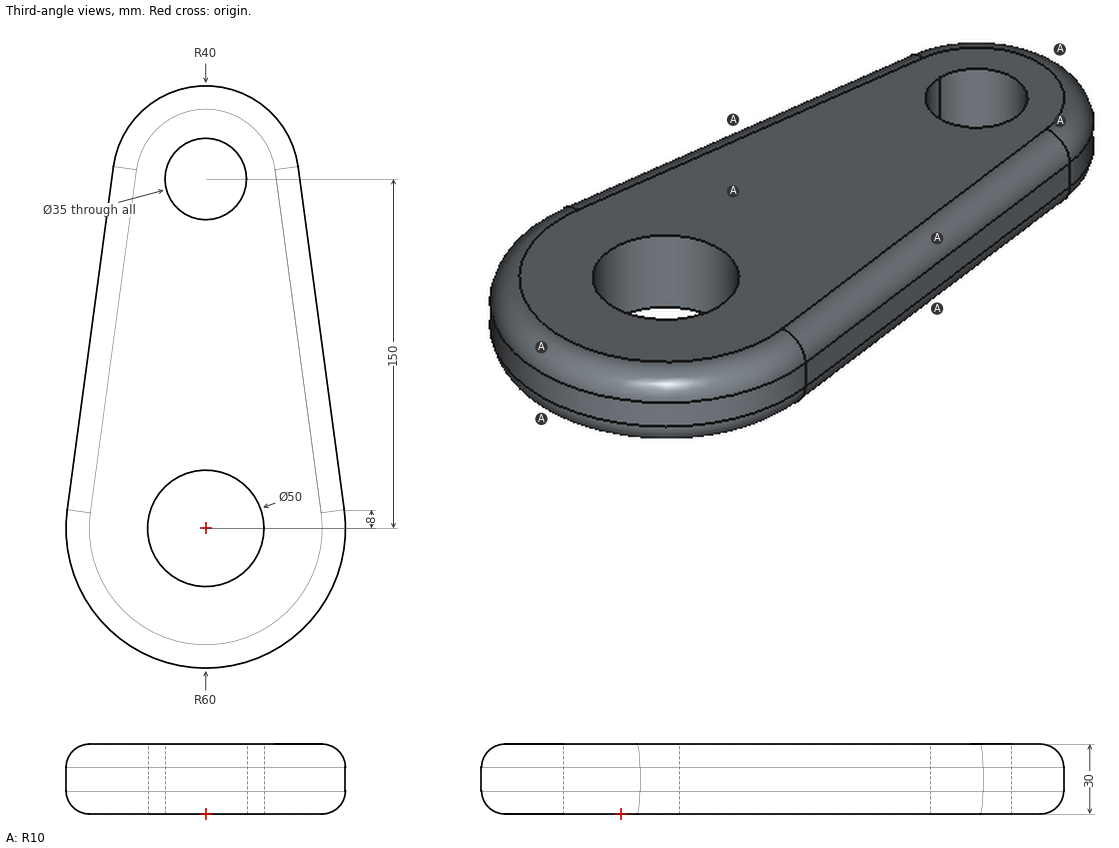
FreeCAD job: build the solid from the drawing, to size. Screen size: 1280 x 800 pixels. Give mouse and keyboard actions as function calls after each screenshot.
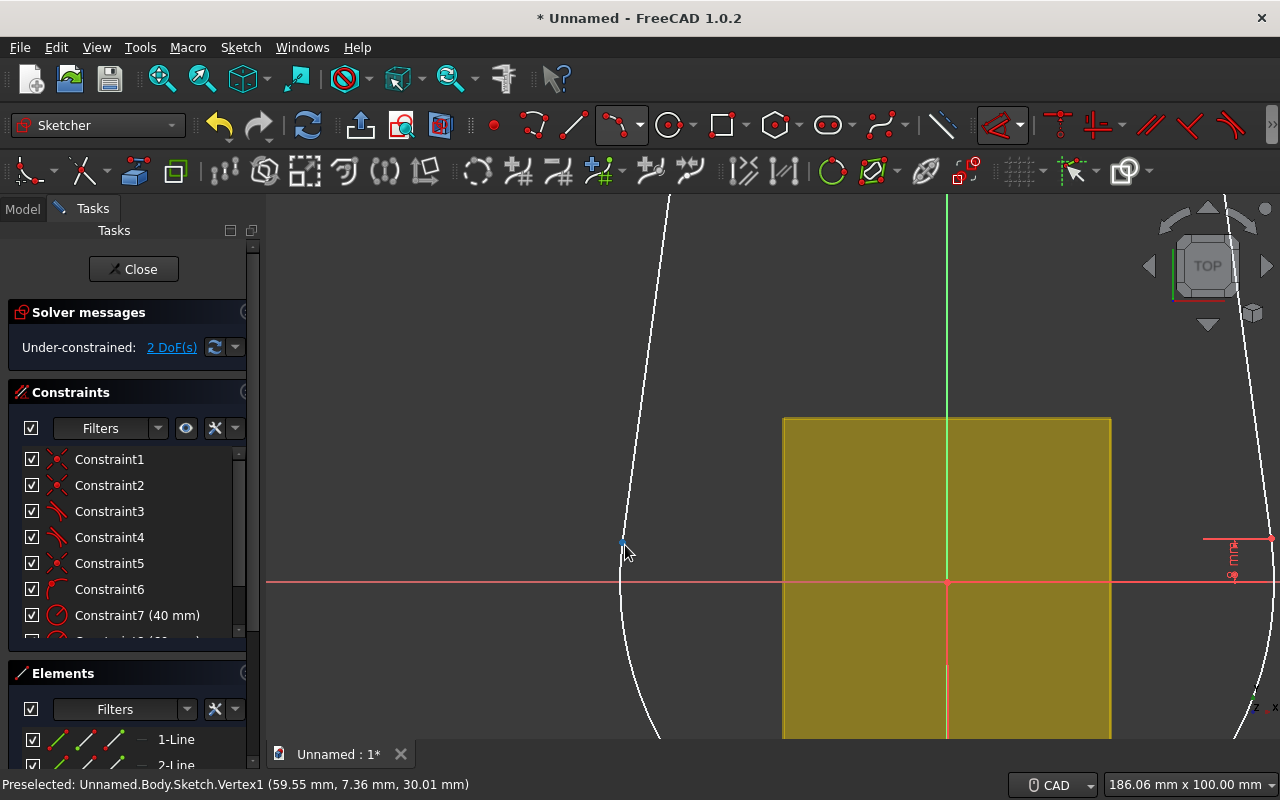
click(623, 542)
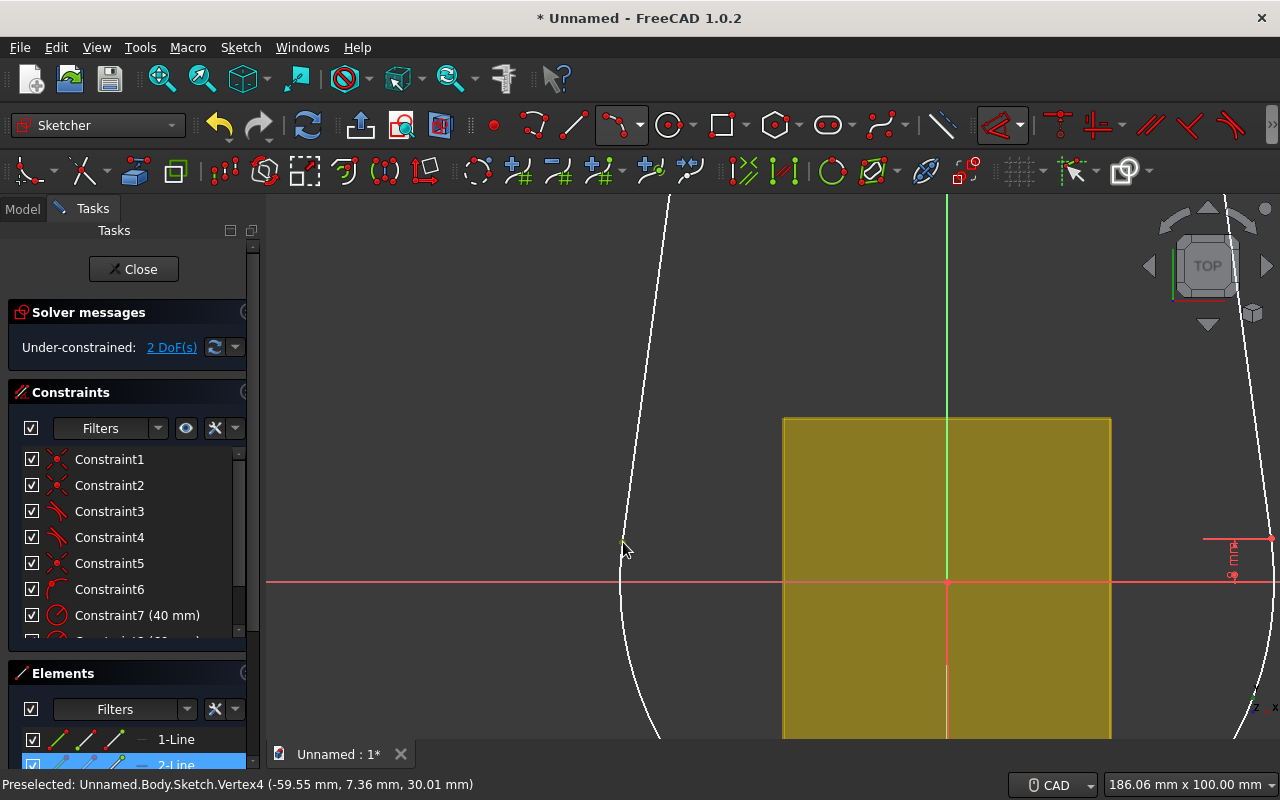
click(1022, 126)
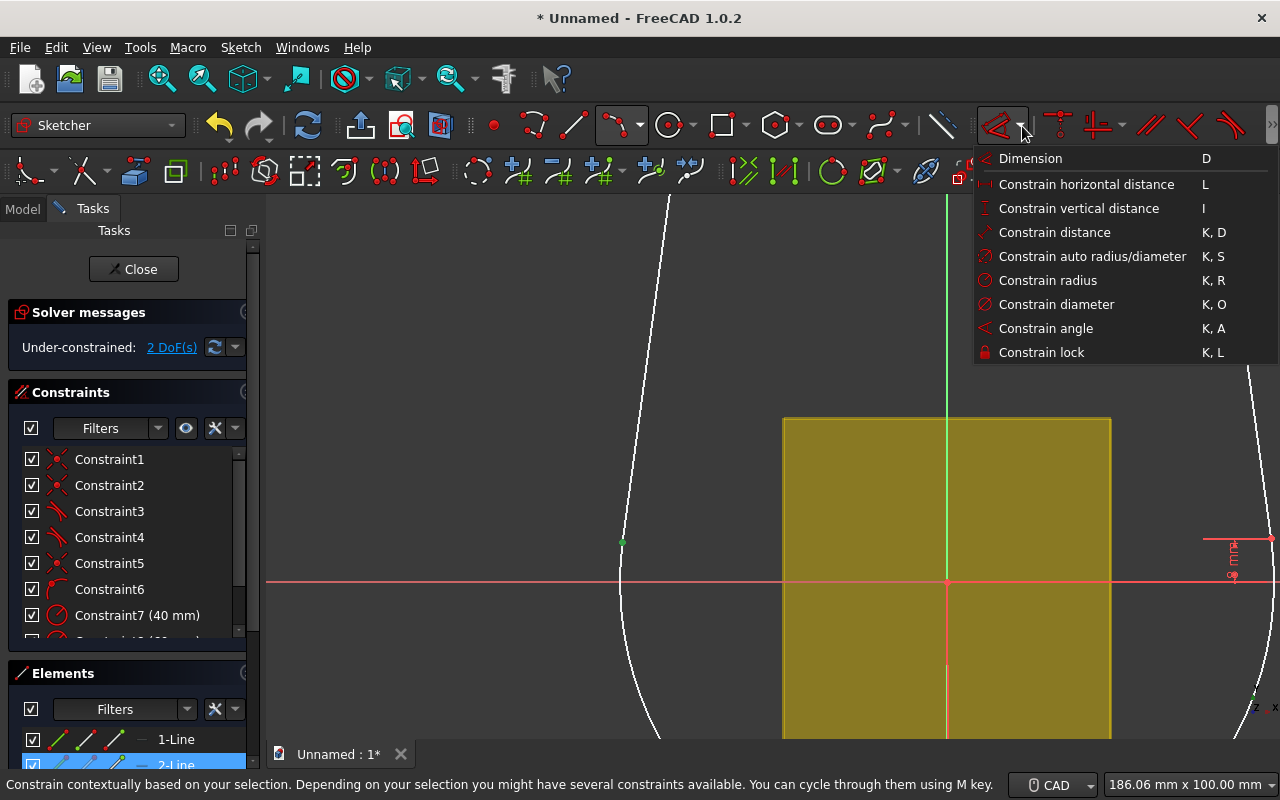
click(1126, 208)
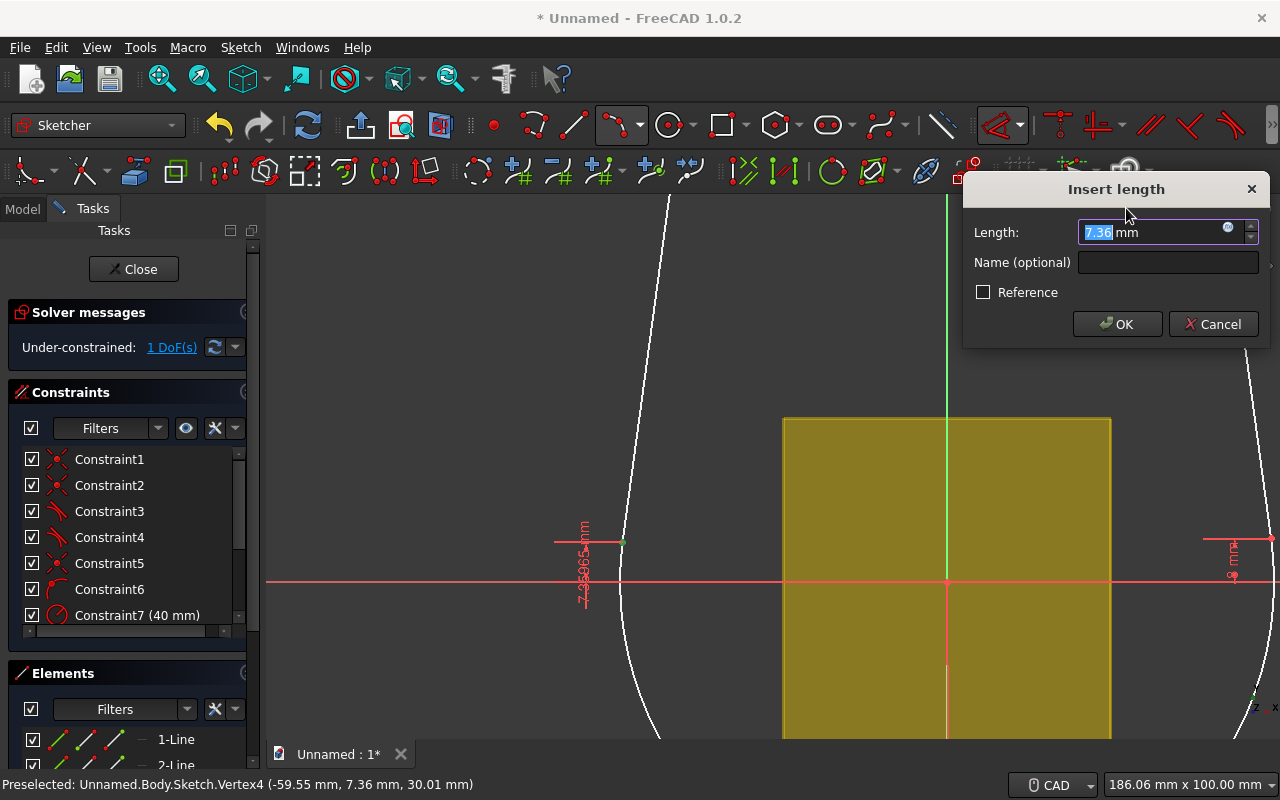
text(8)
key(Return)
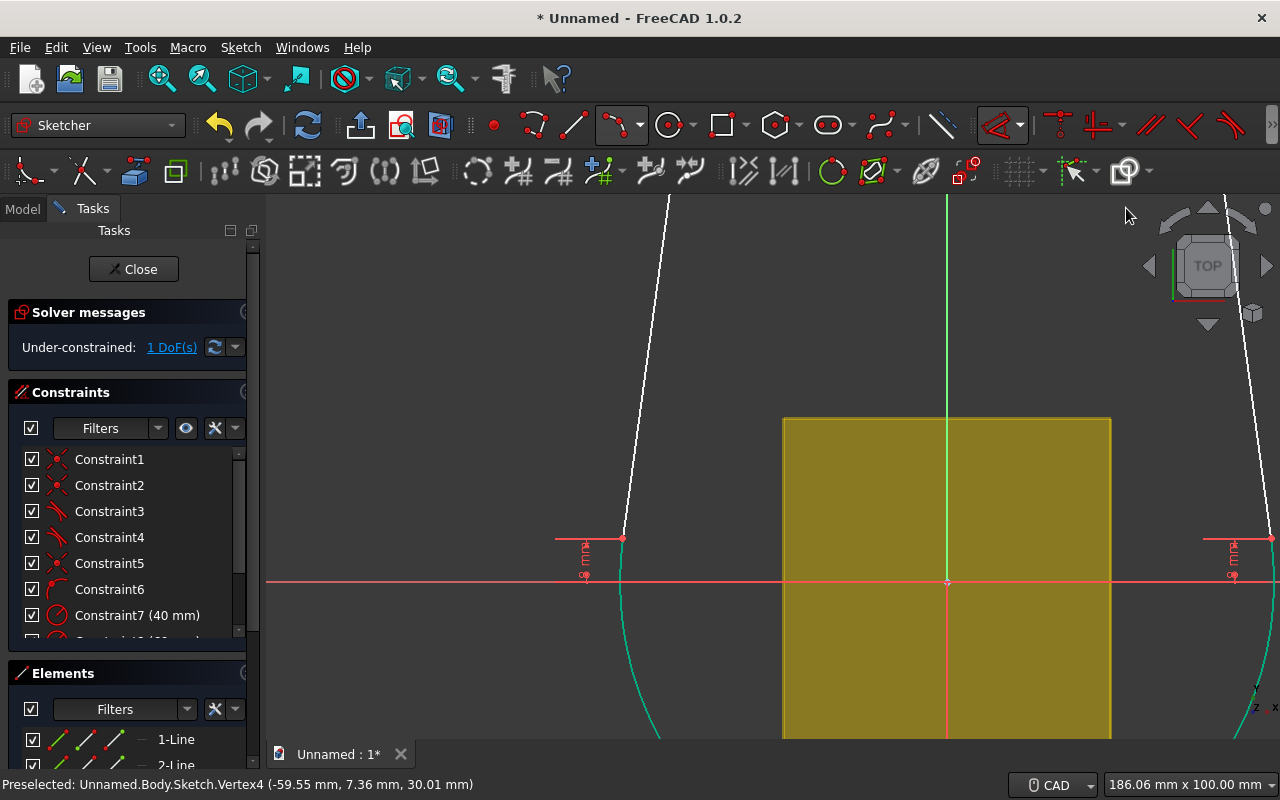
scroll(625, 545, down, 7)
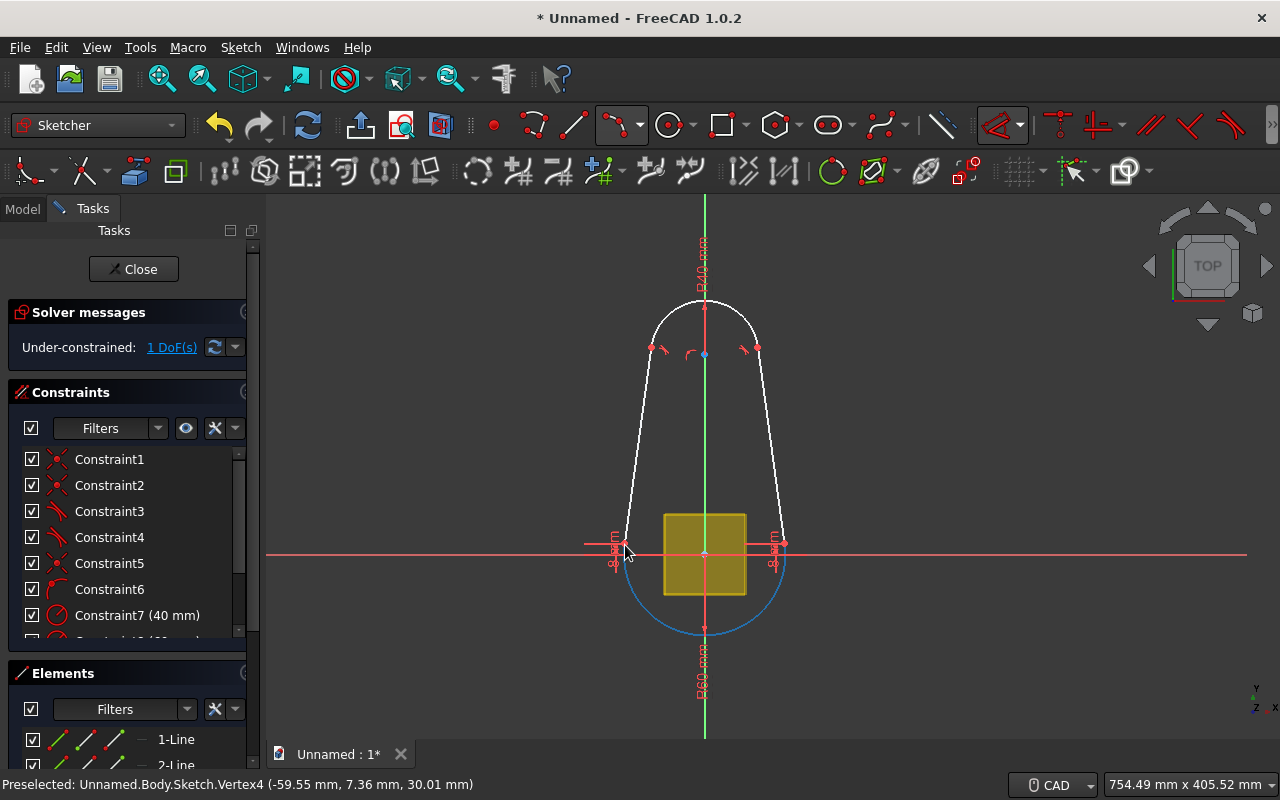
click(705, 355)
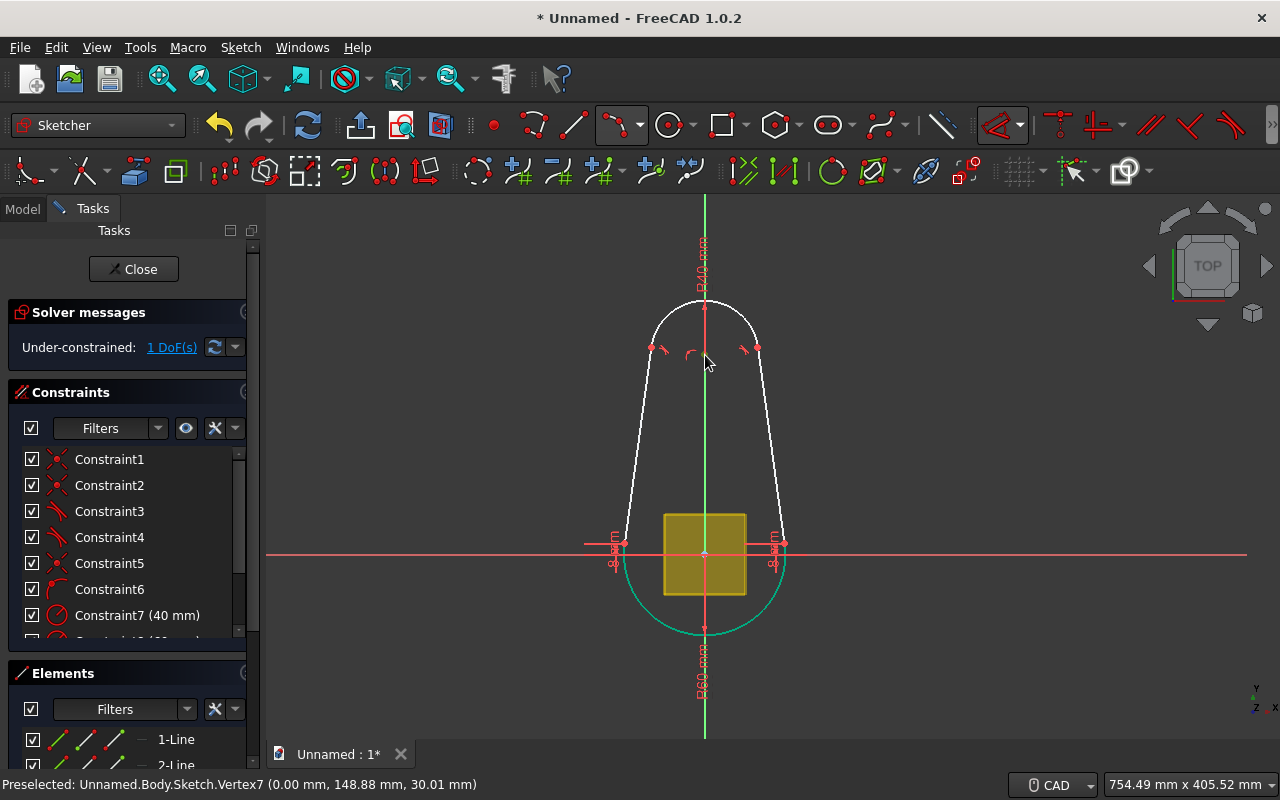
key(i)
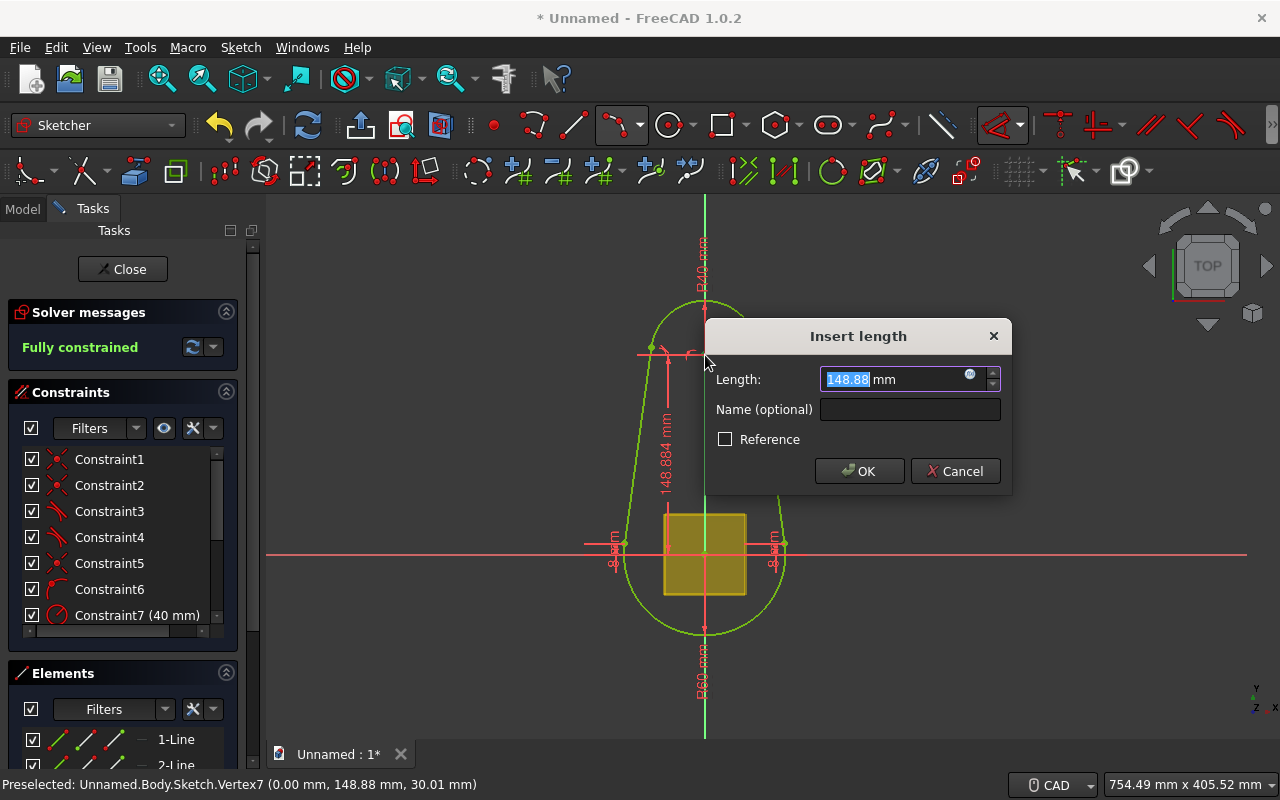
text(150)
key(Return)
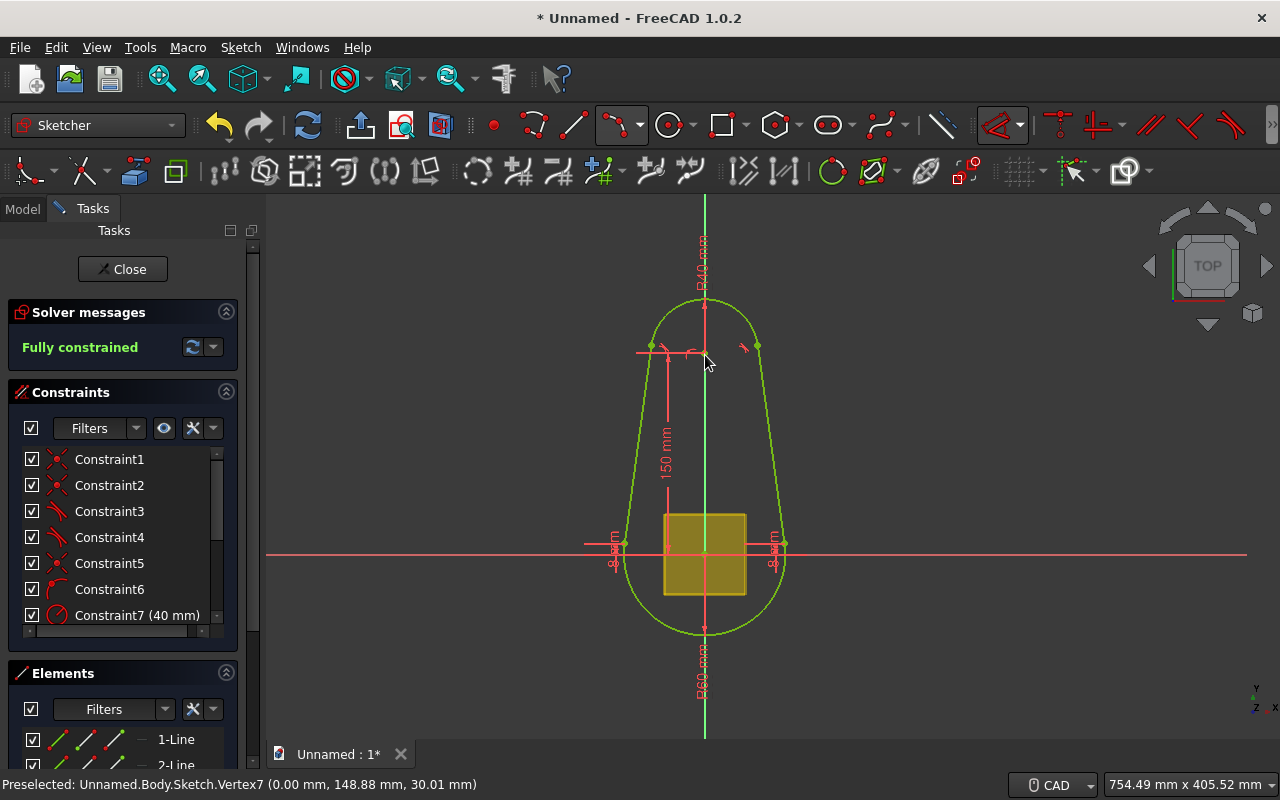
click(123, 269)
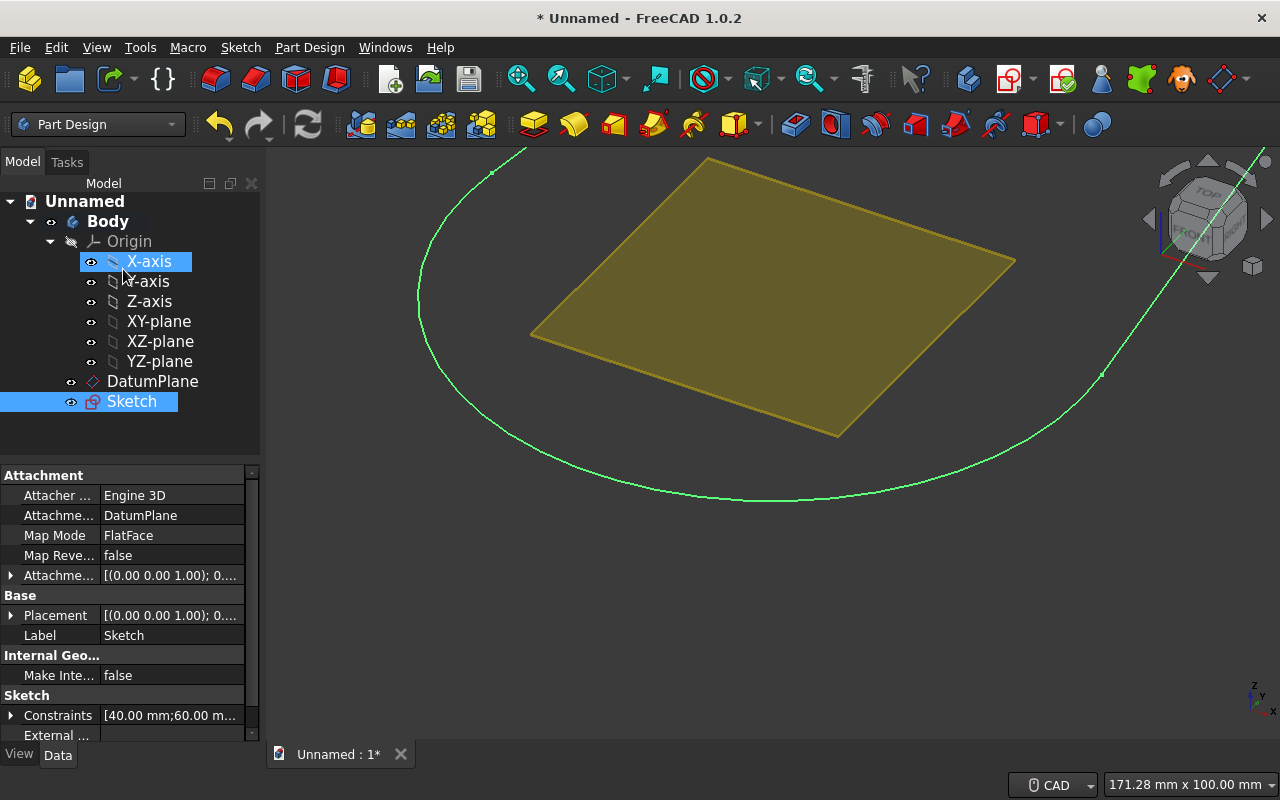
click(534, 124)